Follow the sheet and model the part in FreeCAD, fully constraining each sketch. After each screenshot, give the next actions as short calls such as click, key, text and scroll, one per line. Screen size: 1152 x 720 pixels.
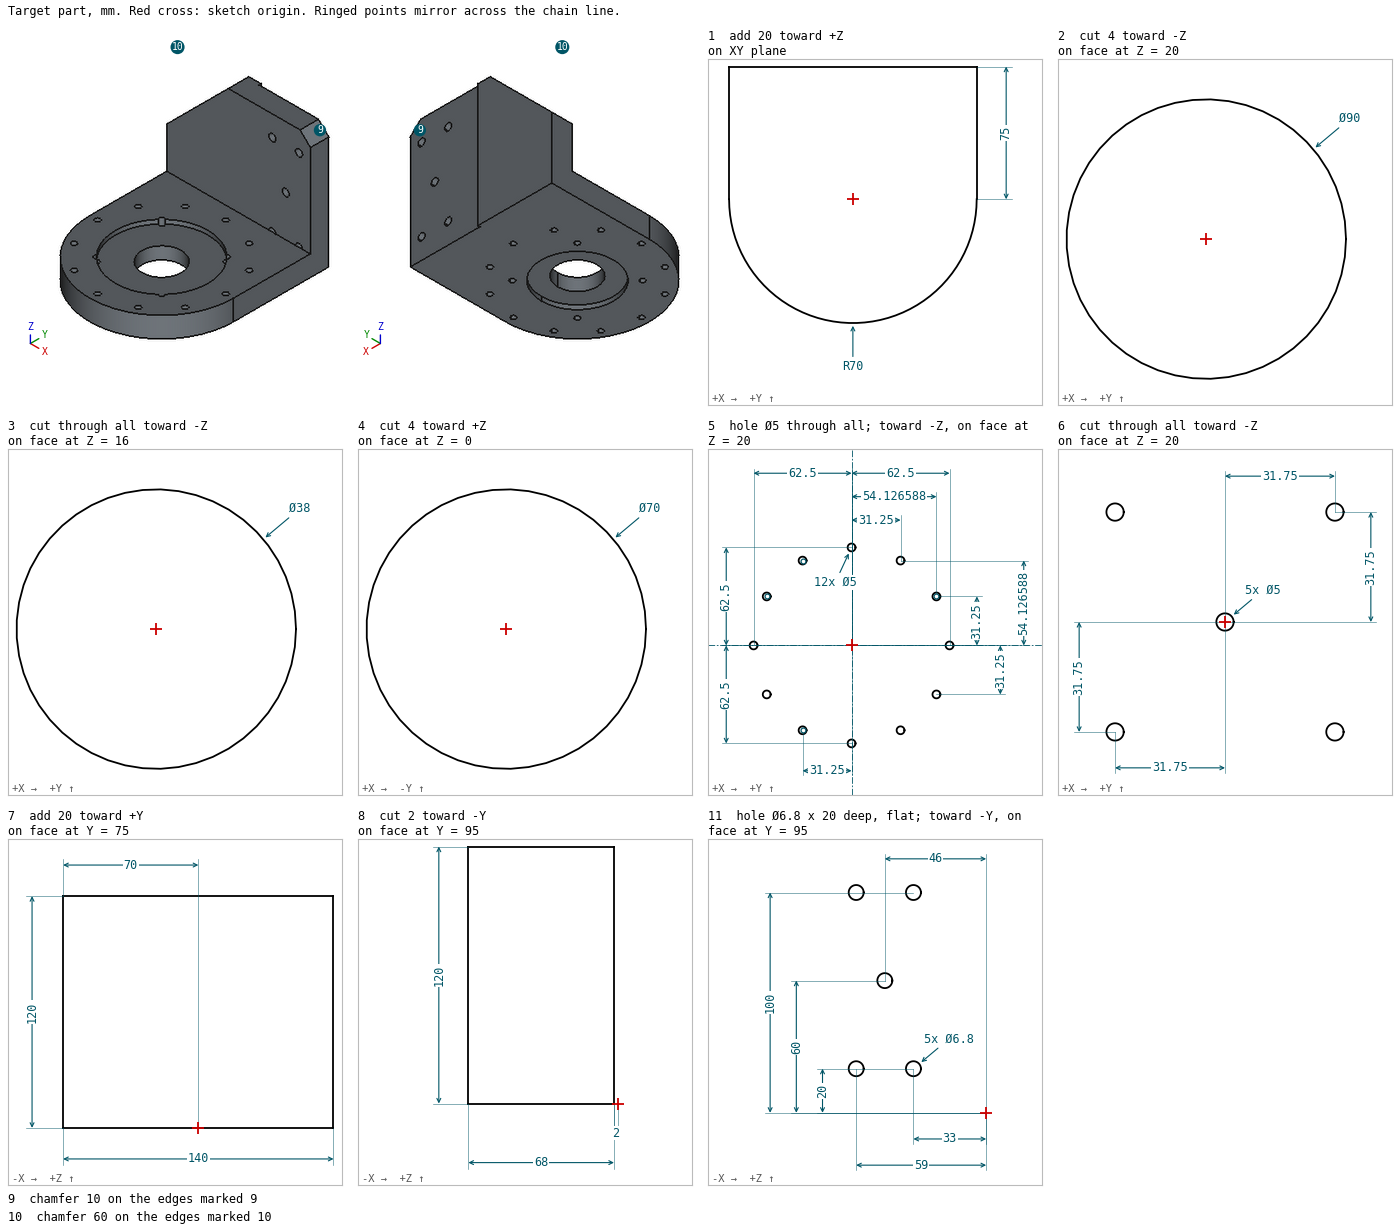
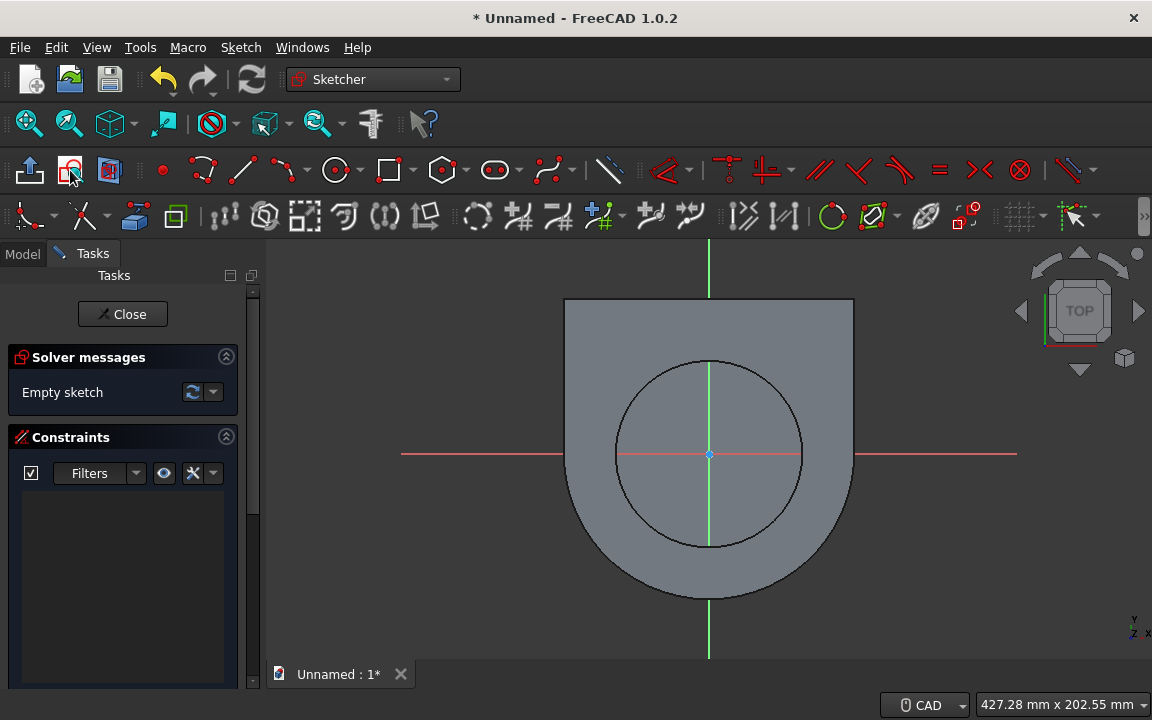
click(110, 170)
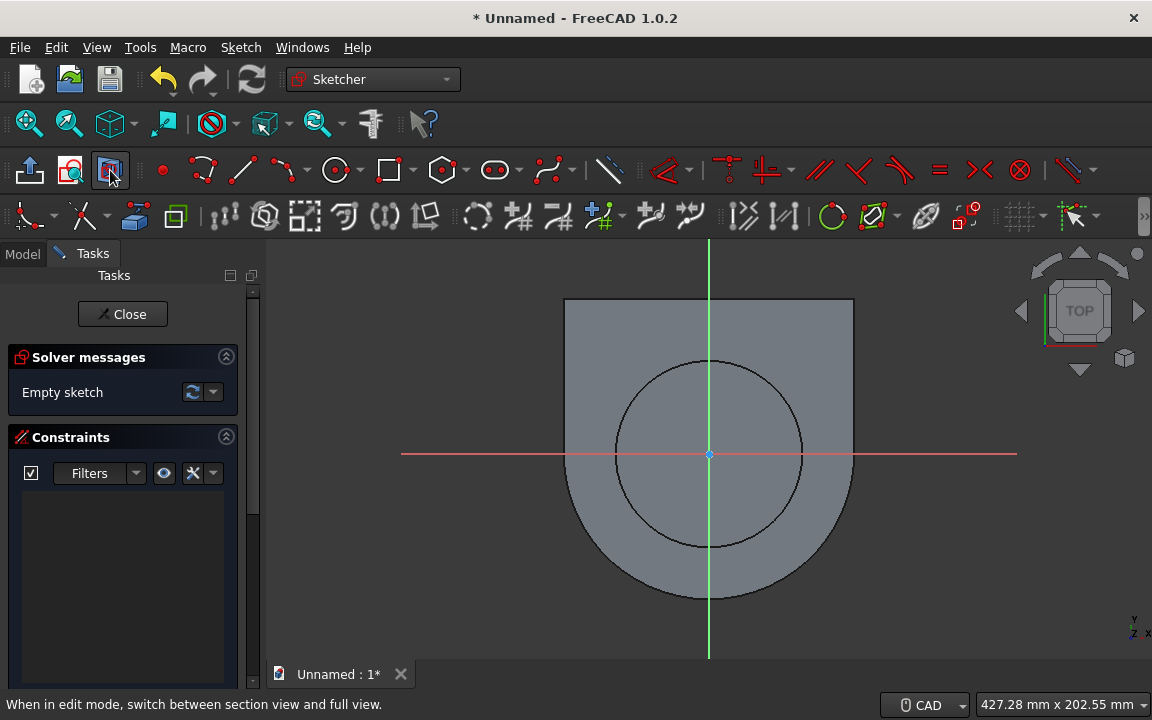
scroll(739, 456, up, 6)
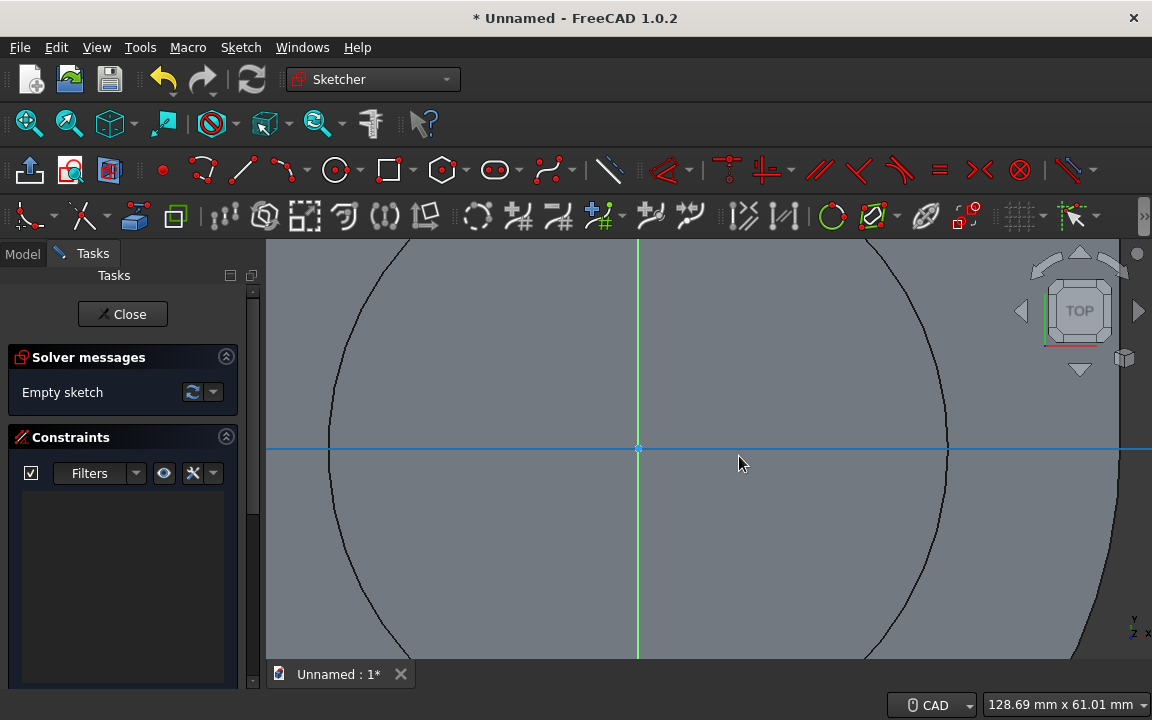
key(g)
key(c)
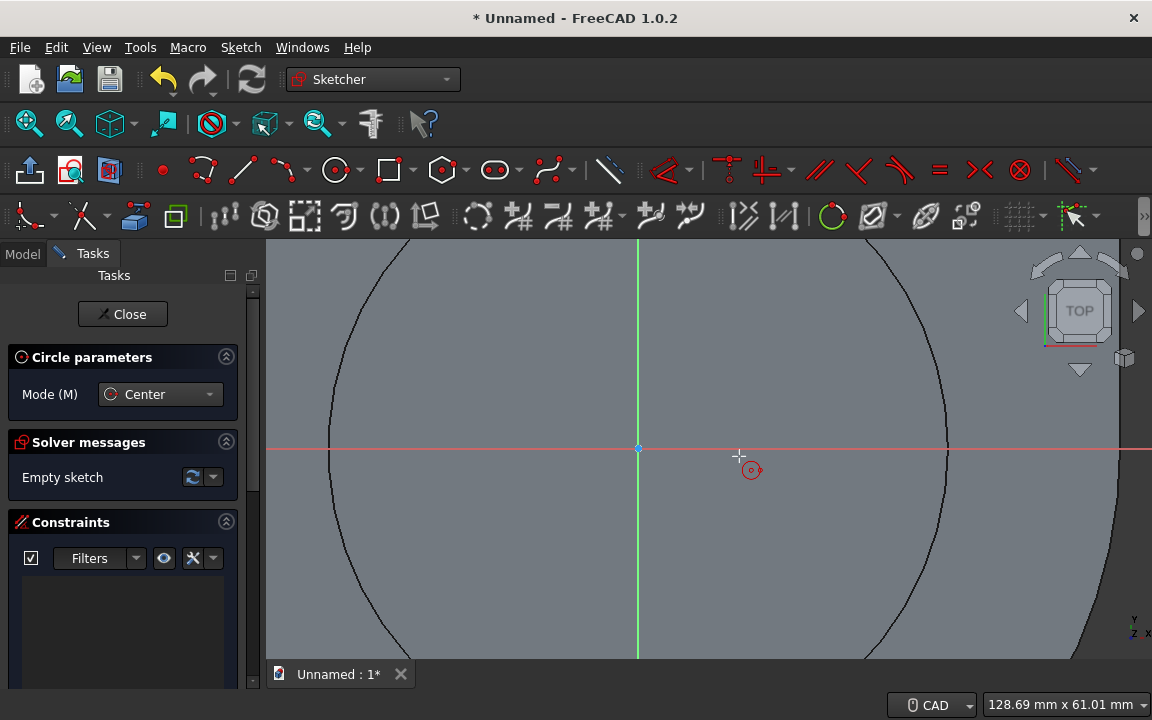
click(638, 449)
move(731, 356)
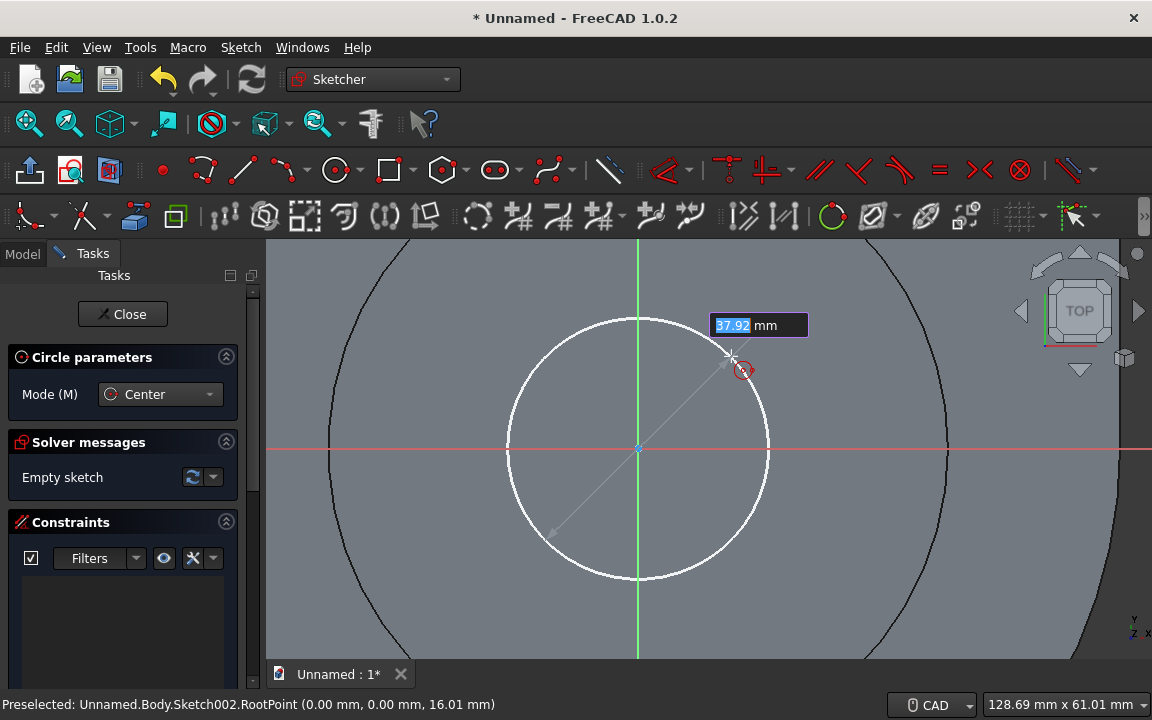
text(38)
key(Return)
key(Escape)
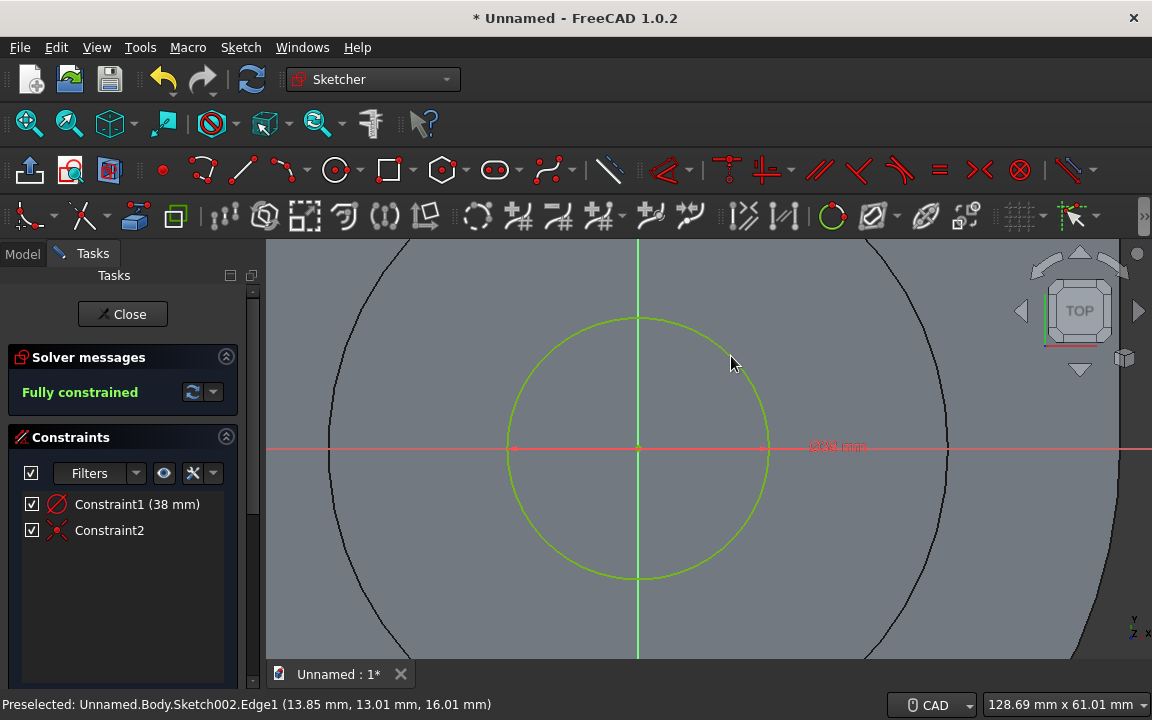
click(123, 314)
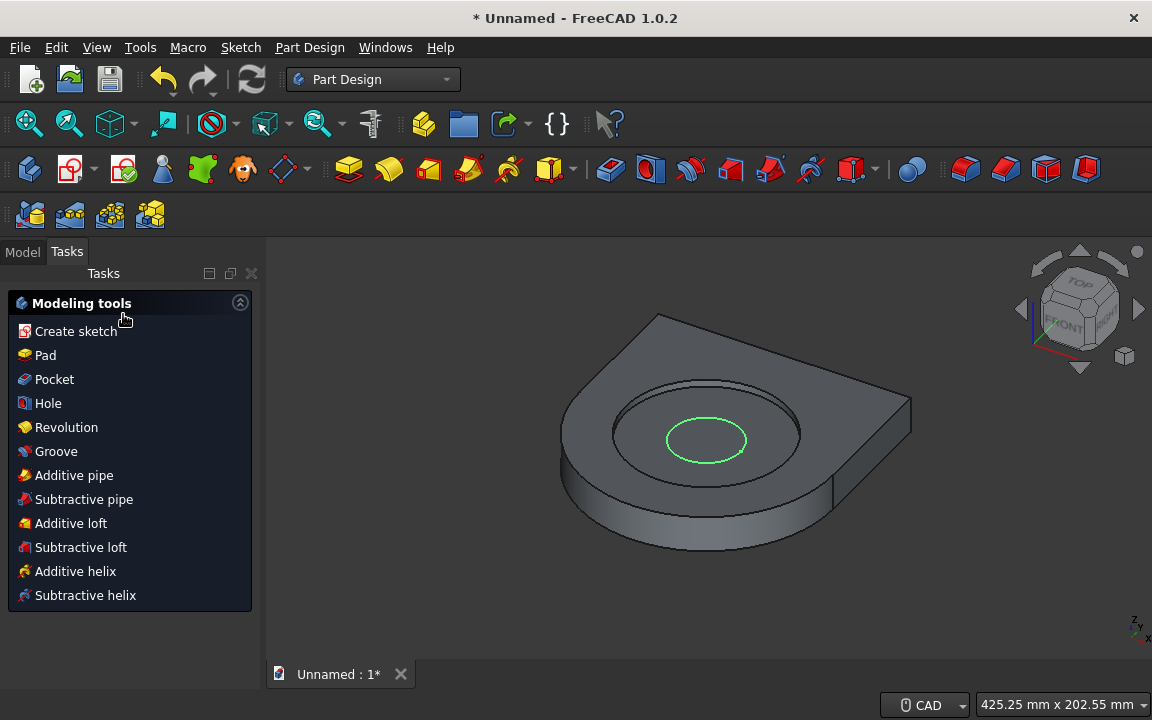
click(612, 170)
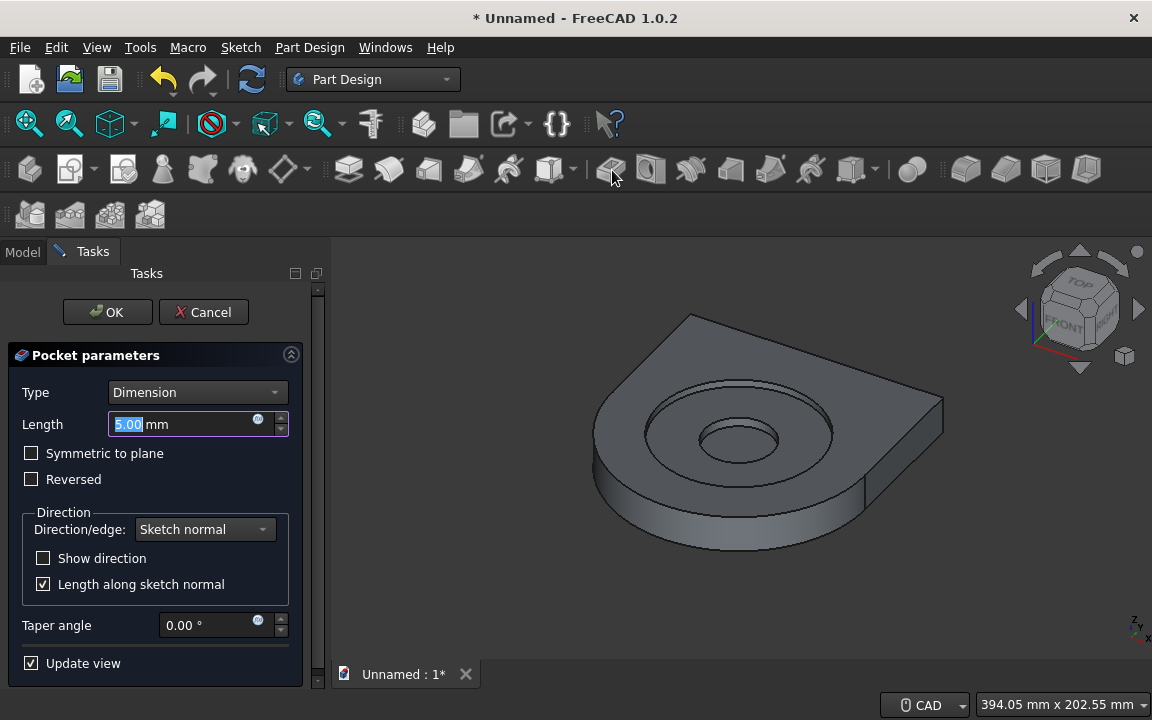
click(198, 392)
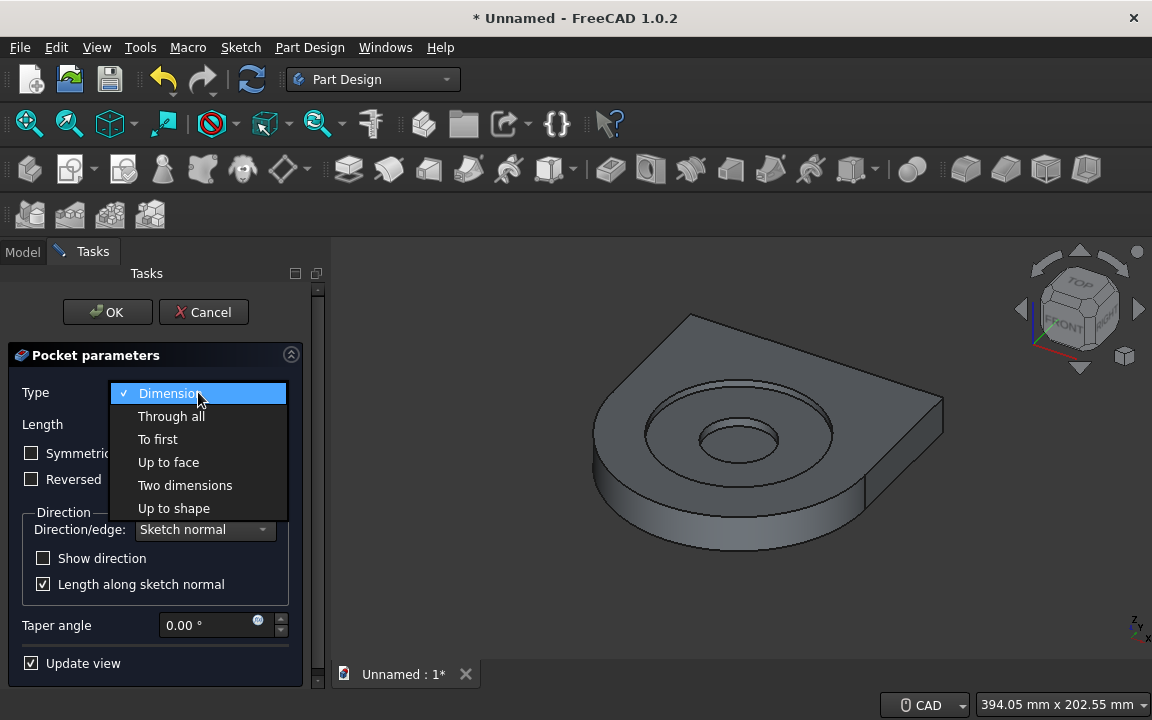
click(198, 416)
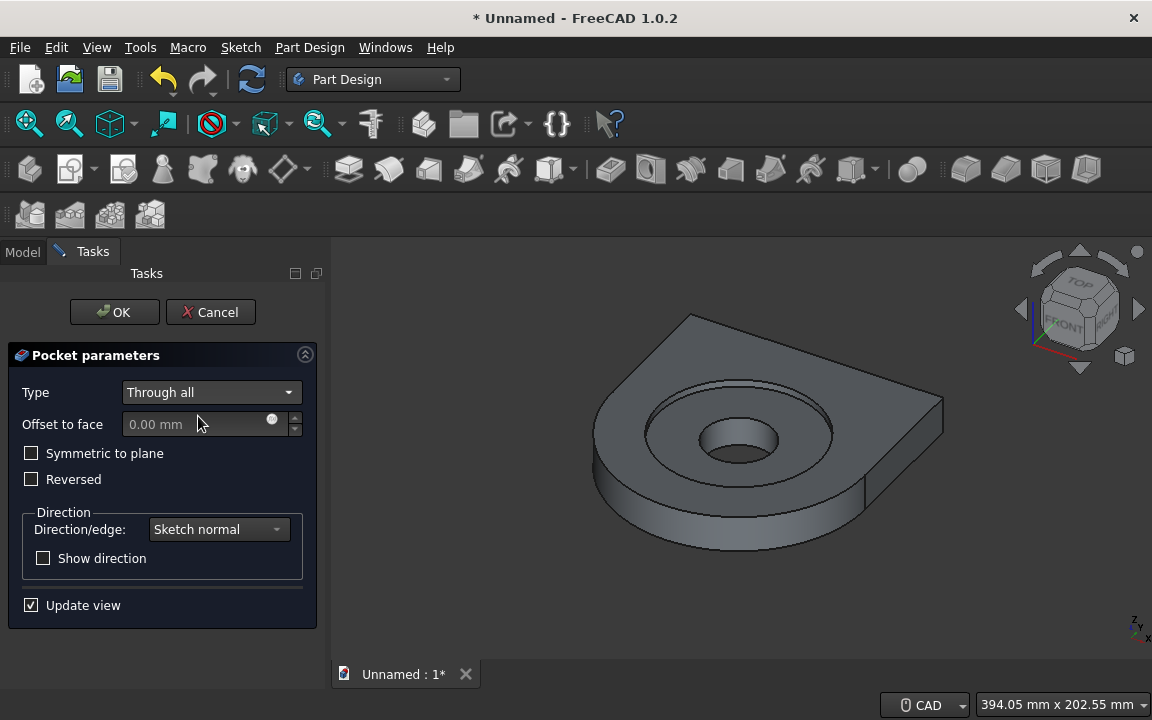
click(115, 312)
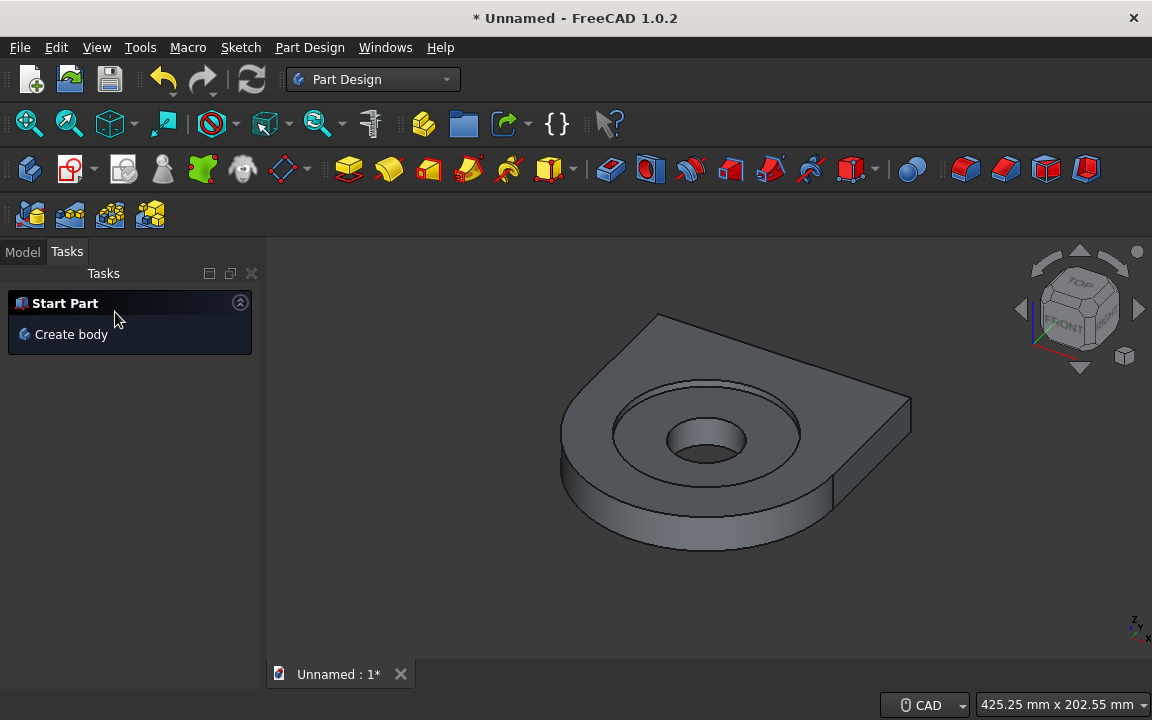
key(5)